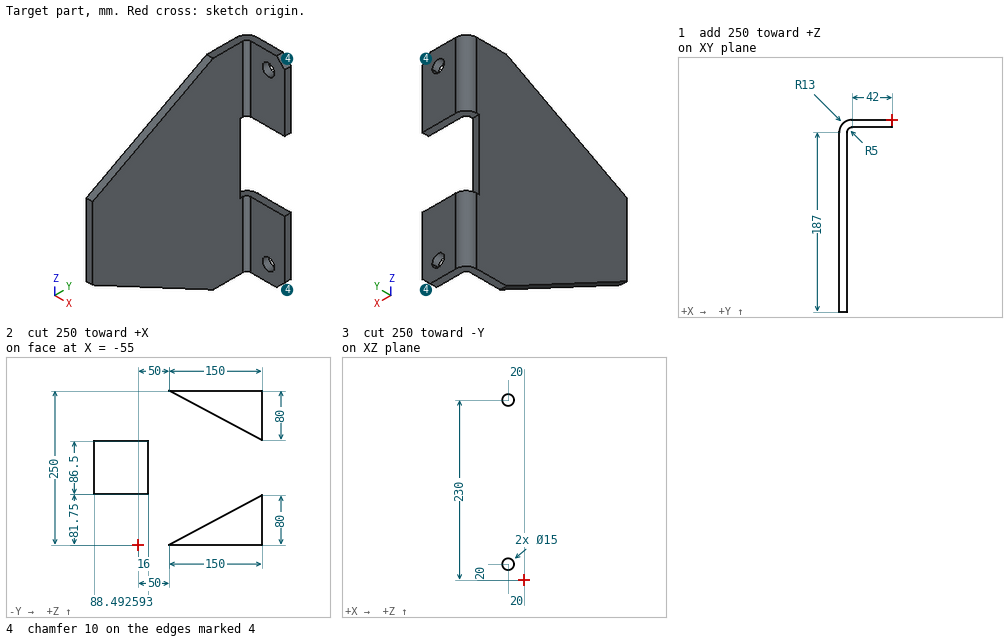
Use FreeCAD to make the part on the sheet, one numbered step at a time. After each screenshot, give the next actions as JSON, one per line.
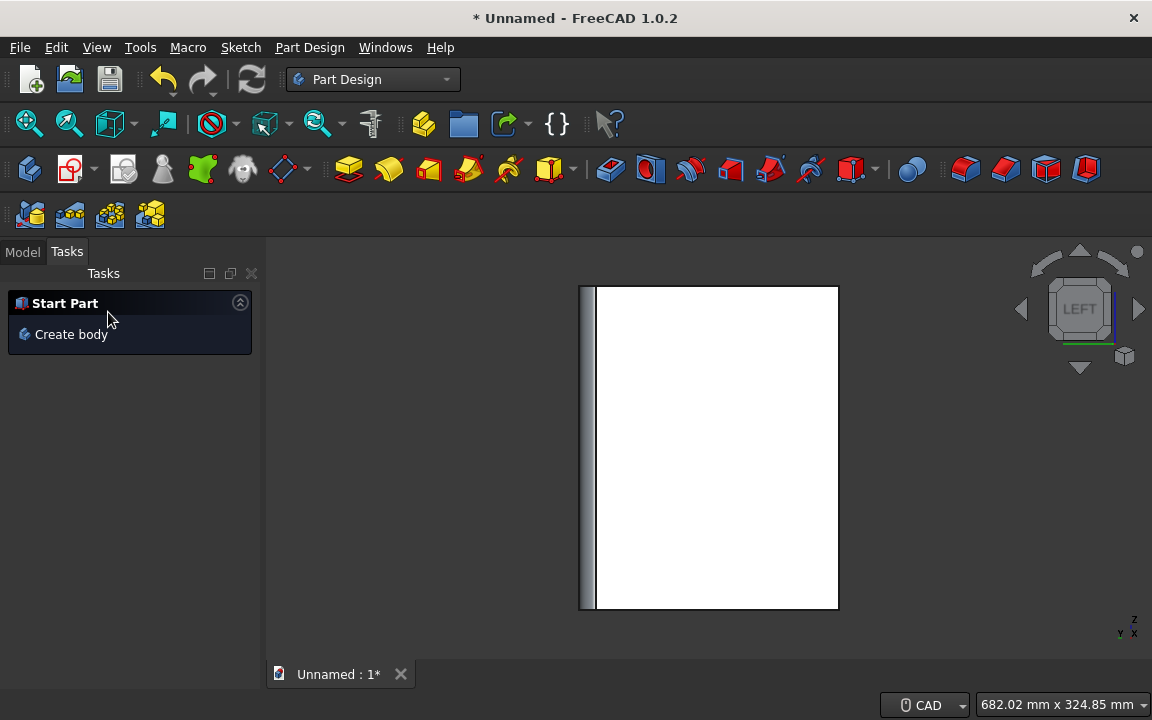
{"action": "left_click", "coordinate": [717, 447]}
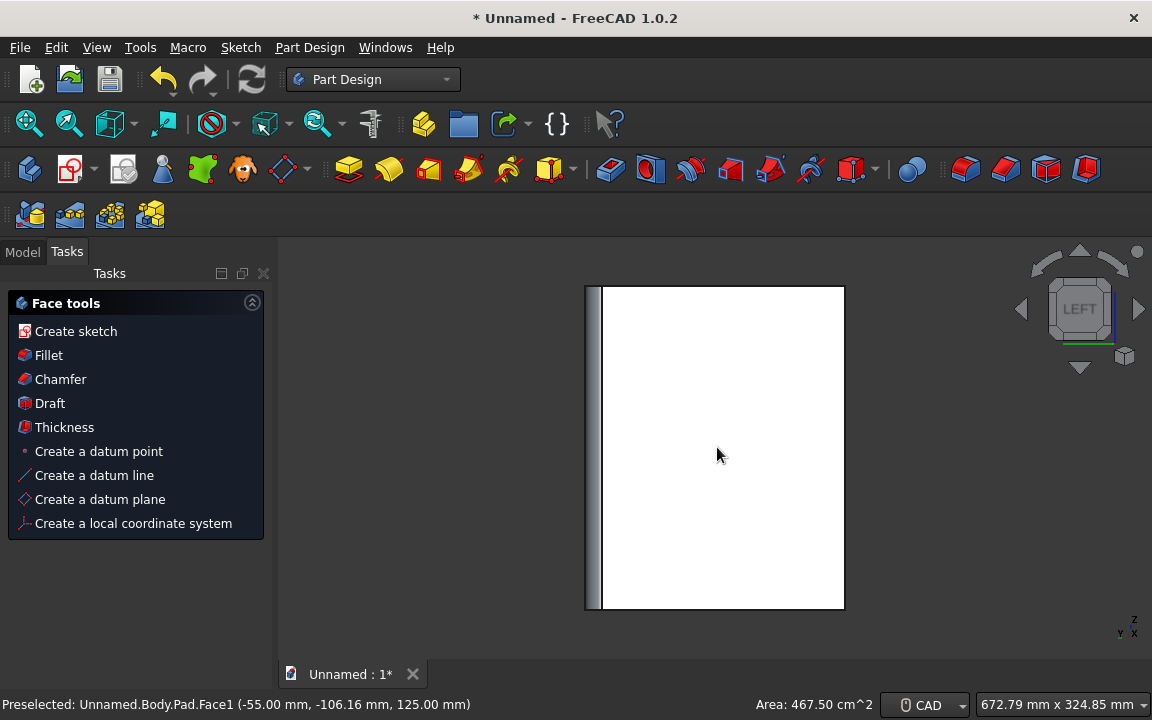
{"action": "left_click", "coordinate": [70, 170]}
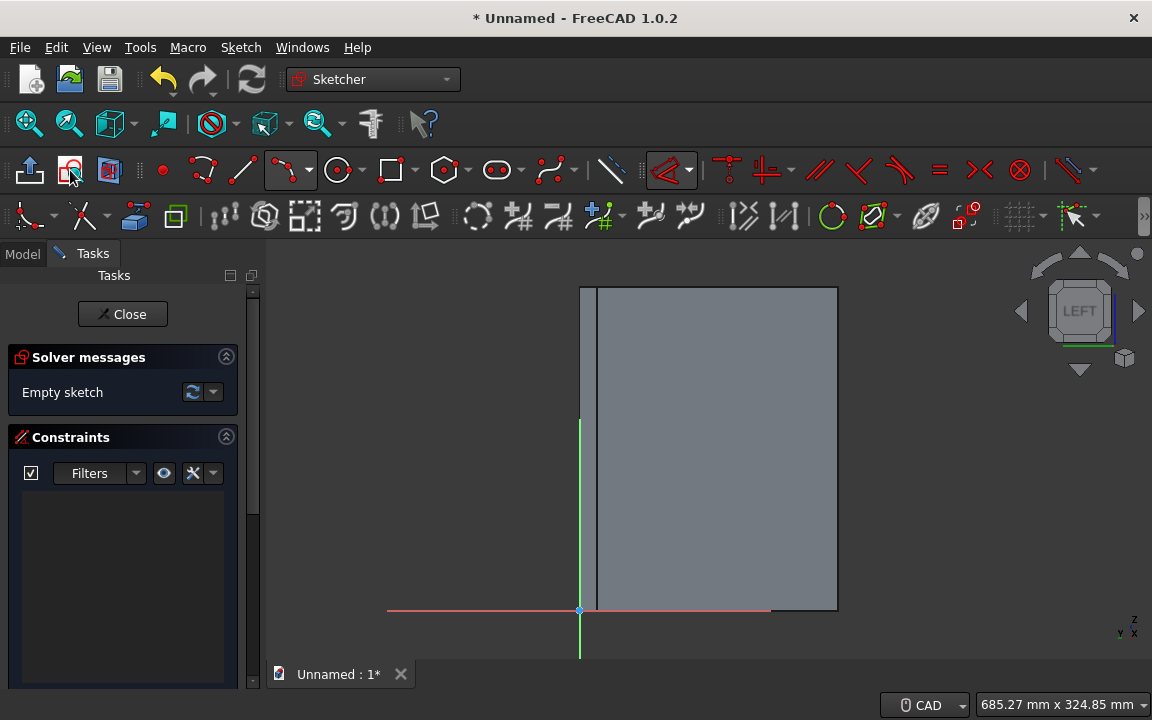
{"action": "scroll", "coordinate": [543, 449], "scroll_direction": "down", "scroll_amount": 1}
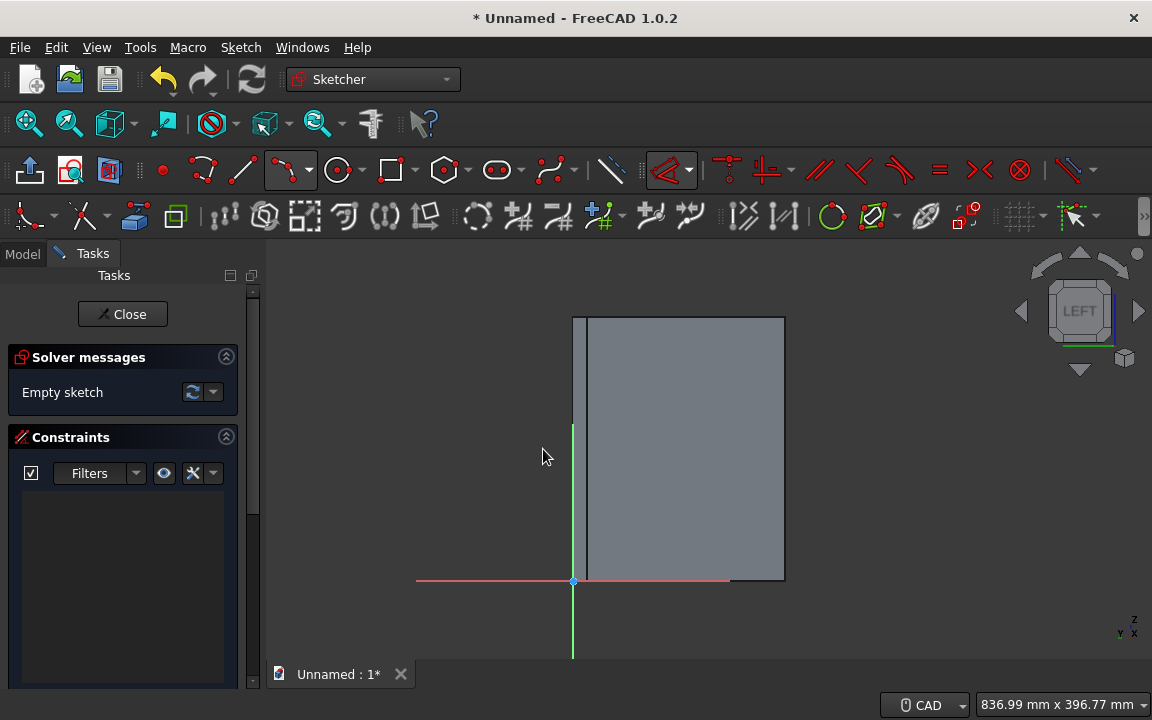
{"action": "left_click", "coordinate": [204, 170]}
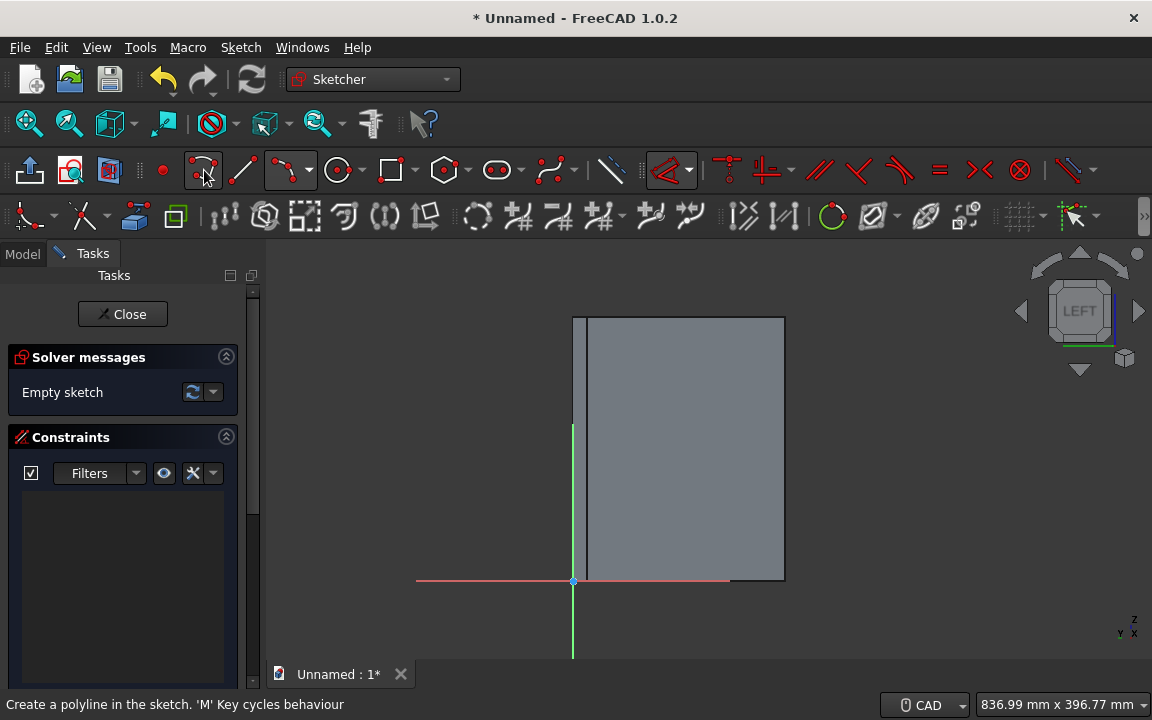
{"action": "left_click", "coordinate": [626, 581]}
{"action": "left_click", "coordinate": [785, 572]}
{"action": "left_click", "coordinate": [785, 497]}
{"action": "left_click", "coordinate": [626, 581]}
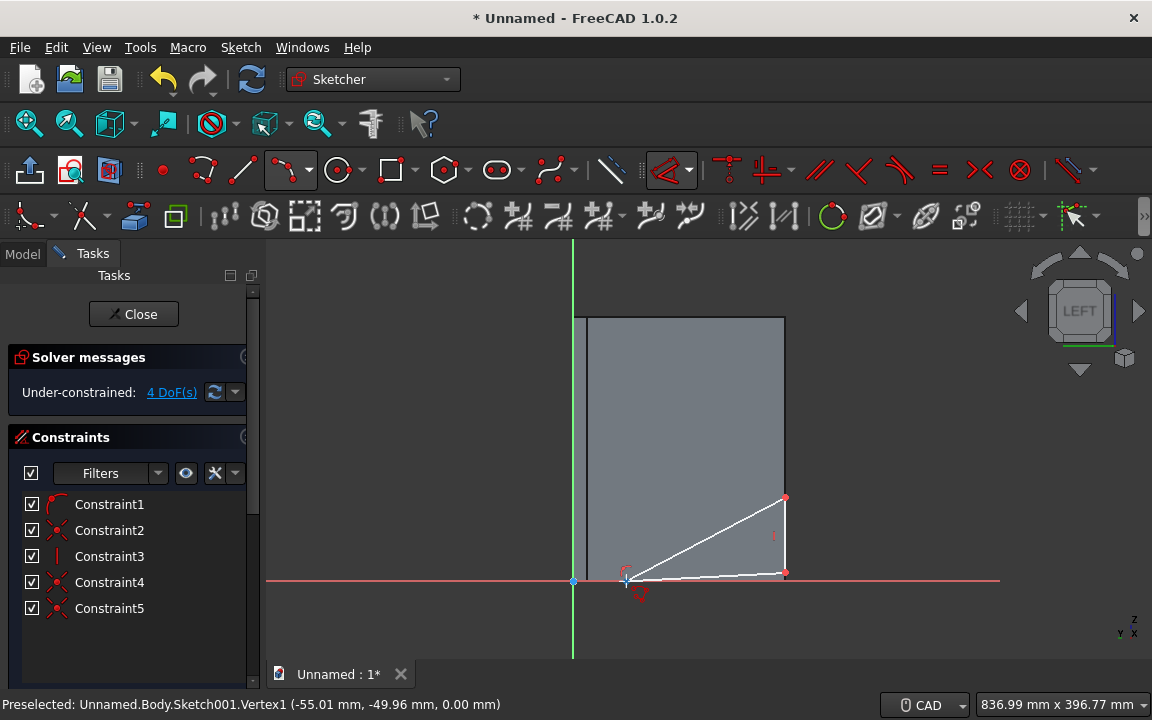
{"action": "left_click", "coordinate": [626, 317]}
{"action": "left_click", "coordinate": [785, 401]}
{"action": "left_click", "coordinate": [785, 317]}
{"action": "left_click", "coordinate": [626, 318]}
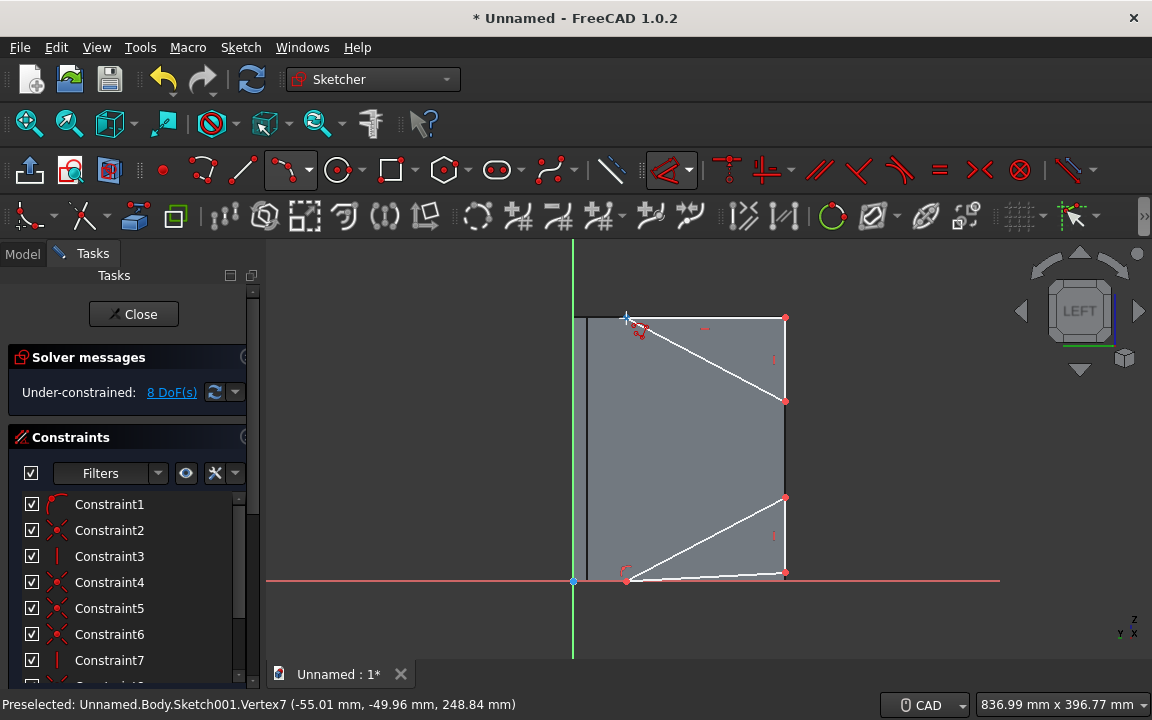
{"action": "left_click", "coordinate": [392, 170]}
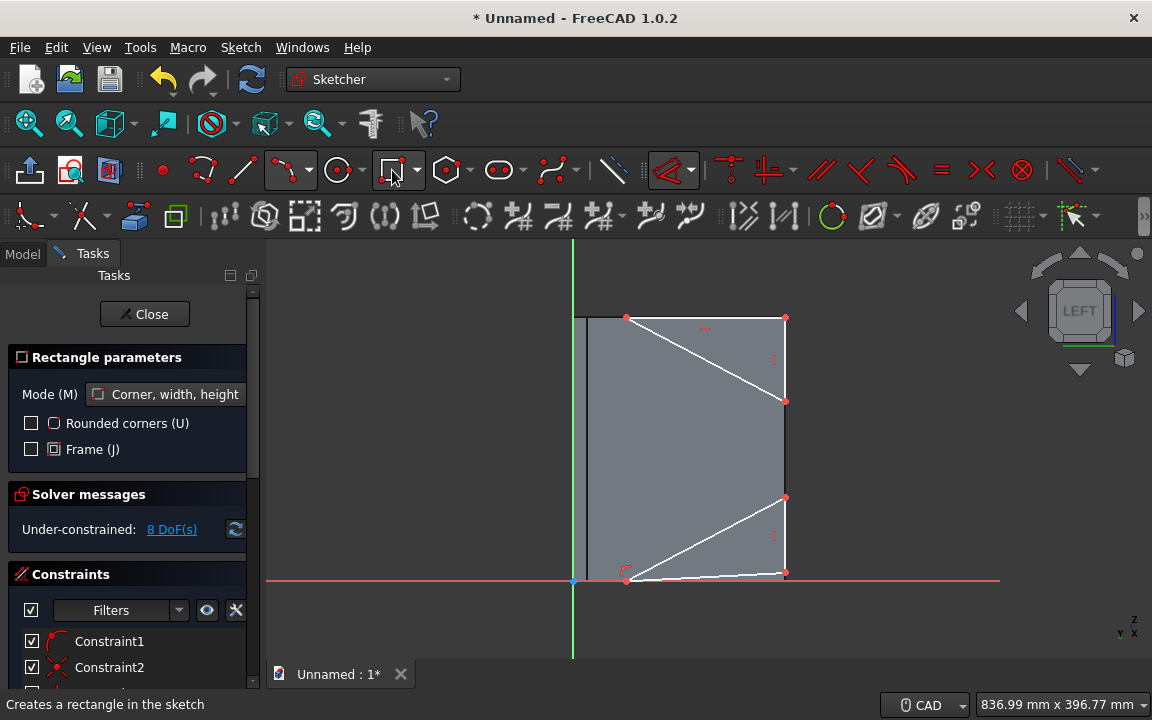
{"action": "left_click", "coordinate": [496, 403]}
{"action": "mouse_move", "coordinate": [590, 495]}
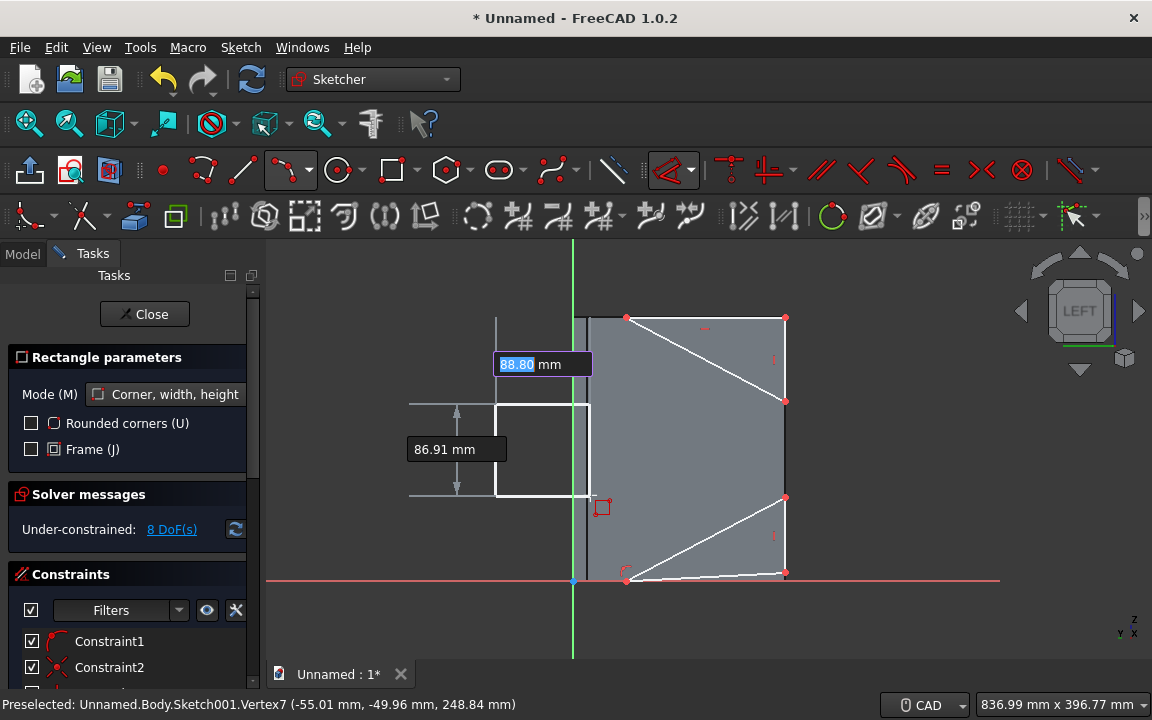
{"action": "type", "text": "88.492593"}
{"action": "key", "text": "Tab"}
{"action": "type", "text": "86.5"}
{"action": "key", "text": "Return"}
{"action": "key", "text": "Escape"}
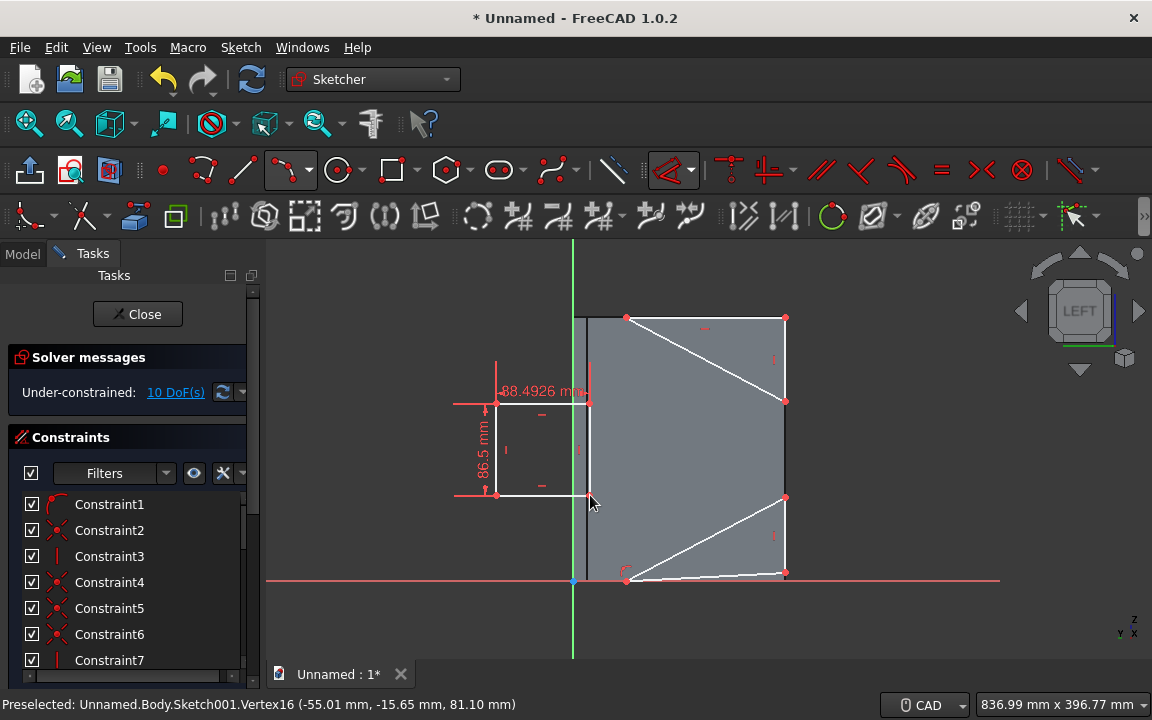
{"action": "left_click", "coordinate": [674, 579]}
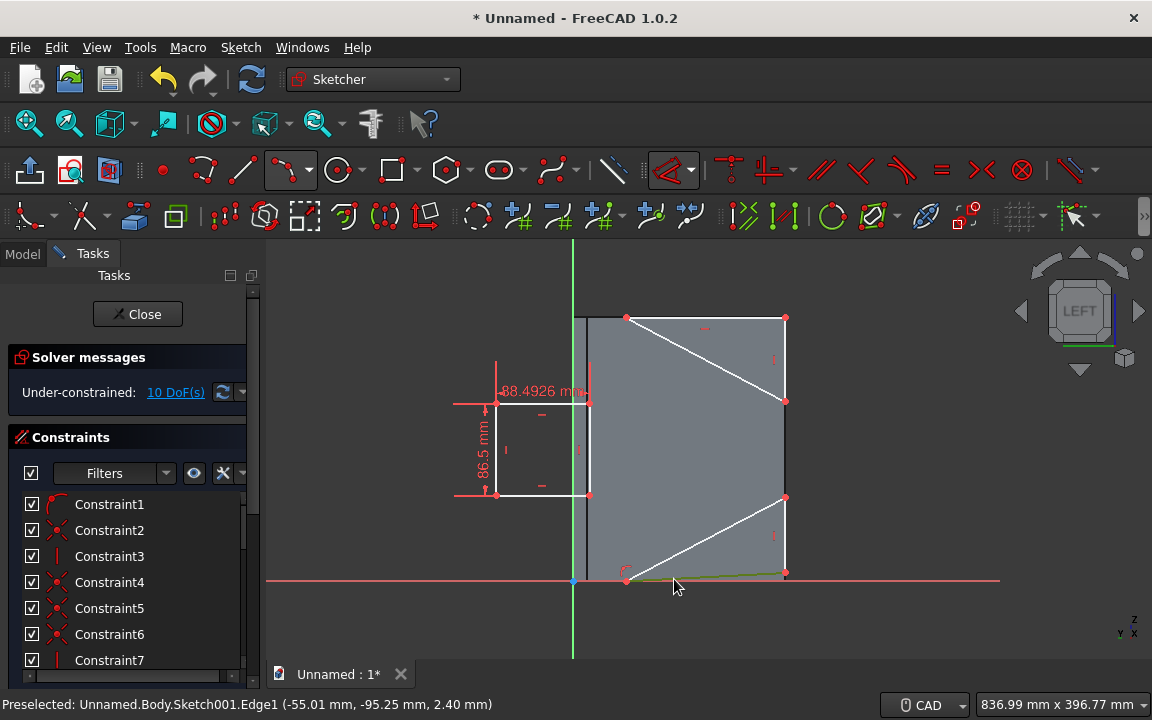
{"action": "left_click", "coordinate": [796, 170]}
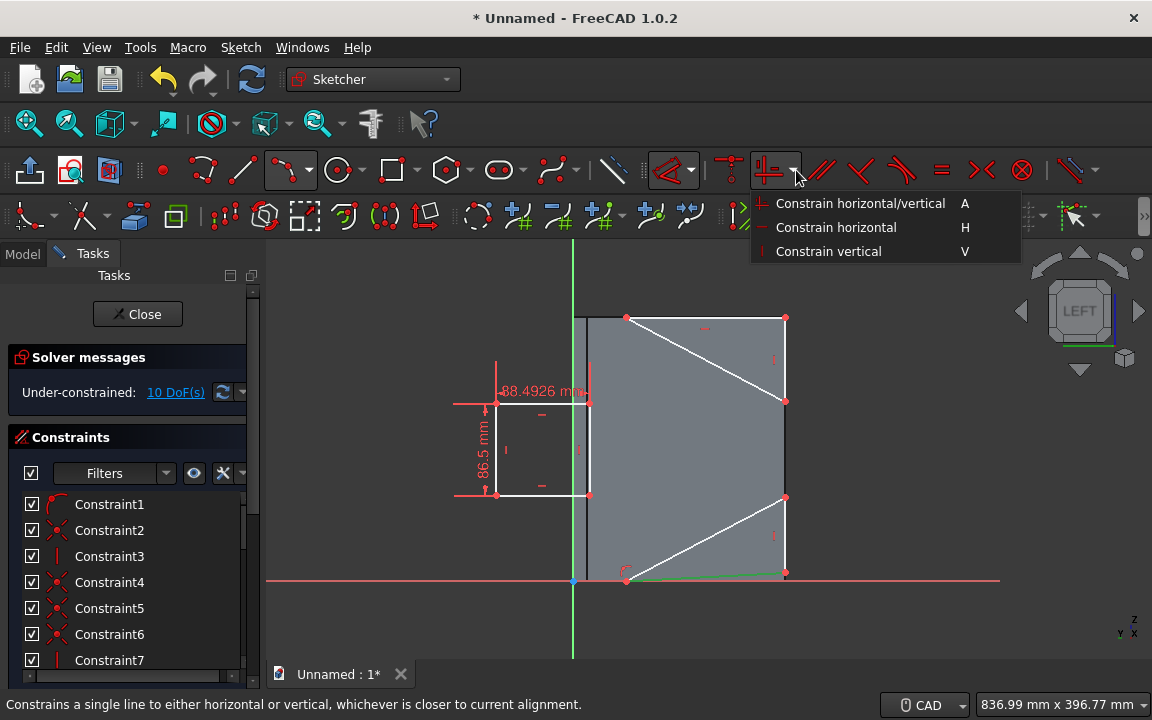
{"action": "left_click", "coordinate": [886, 227]}